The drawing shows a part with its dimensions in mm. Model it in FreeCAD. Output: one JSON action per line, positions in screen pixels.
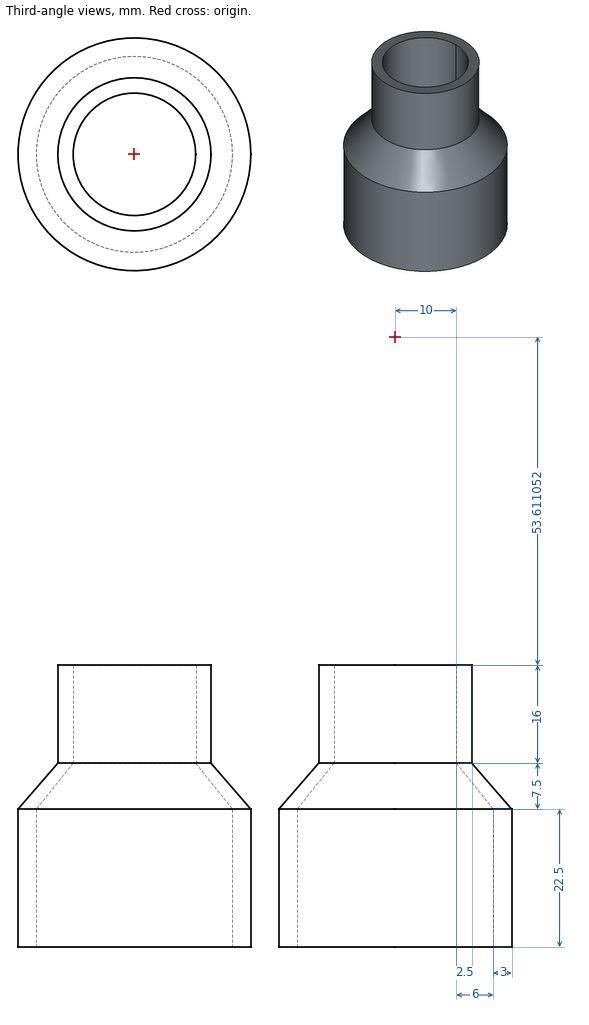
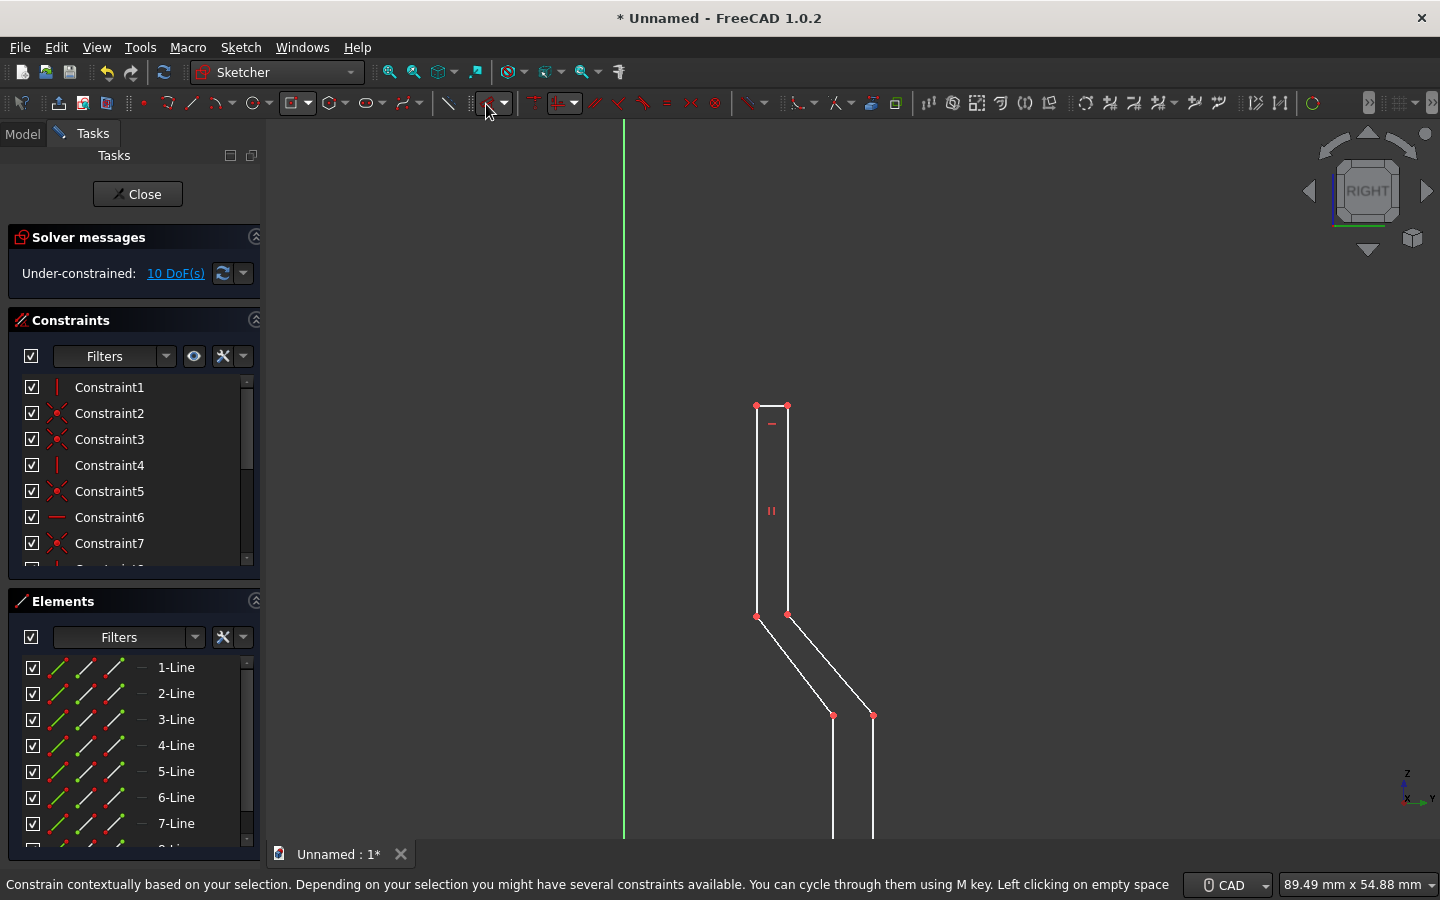
{"action": "scroll", "coordinate": [805, 552], "scroll_direction": "down", "scroll_amount": 5}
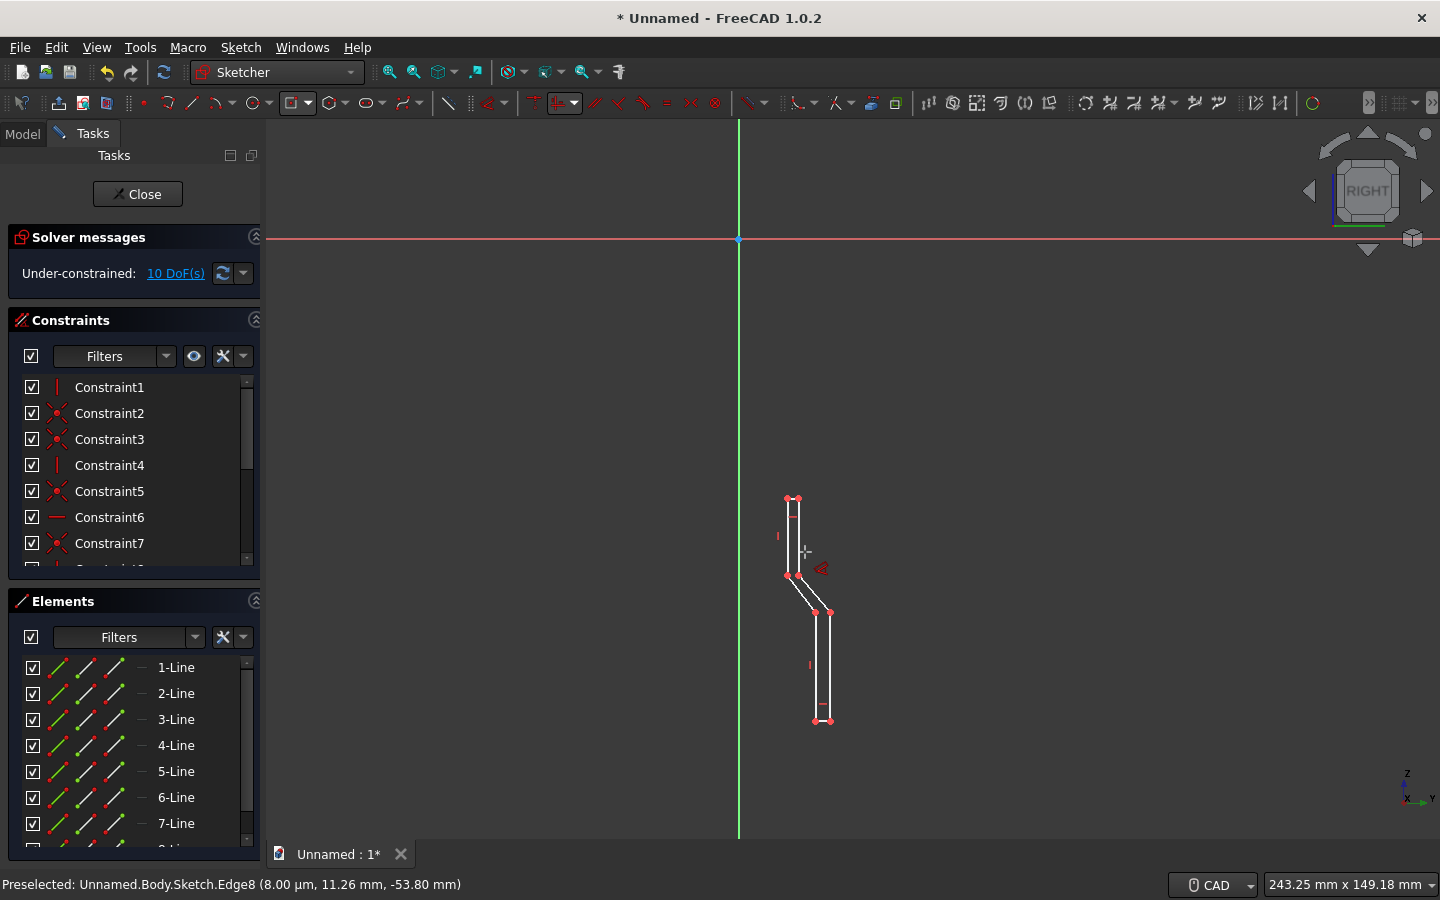
{"action": "scroll", "coordinate": [820, 721], "scroll_direction": "up", "scroll_amount": 6}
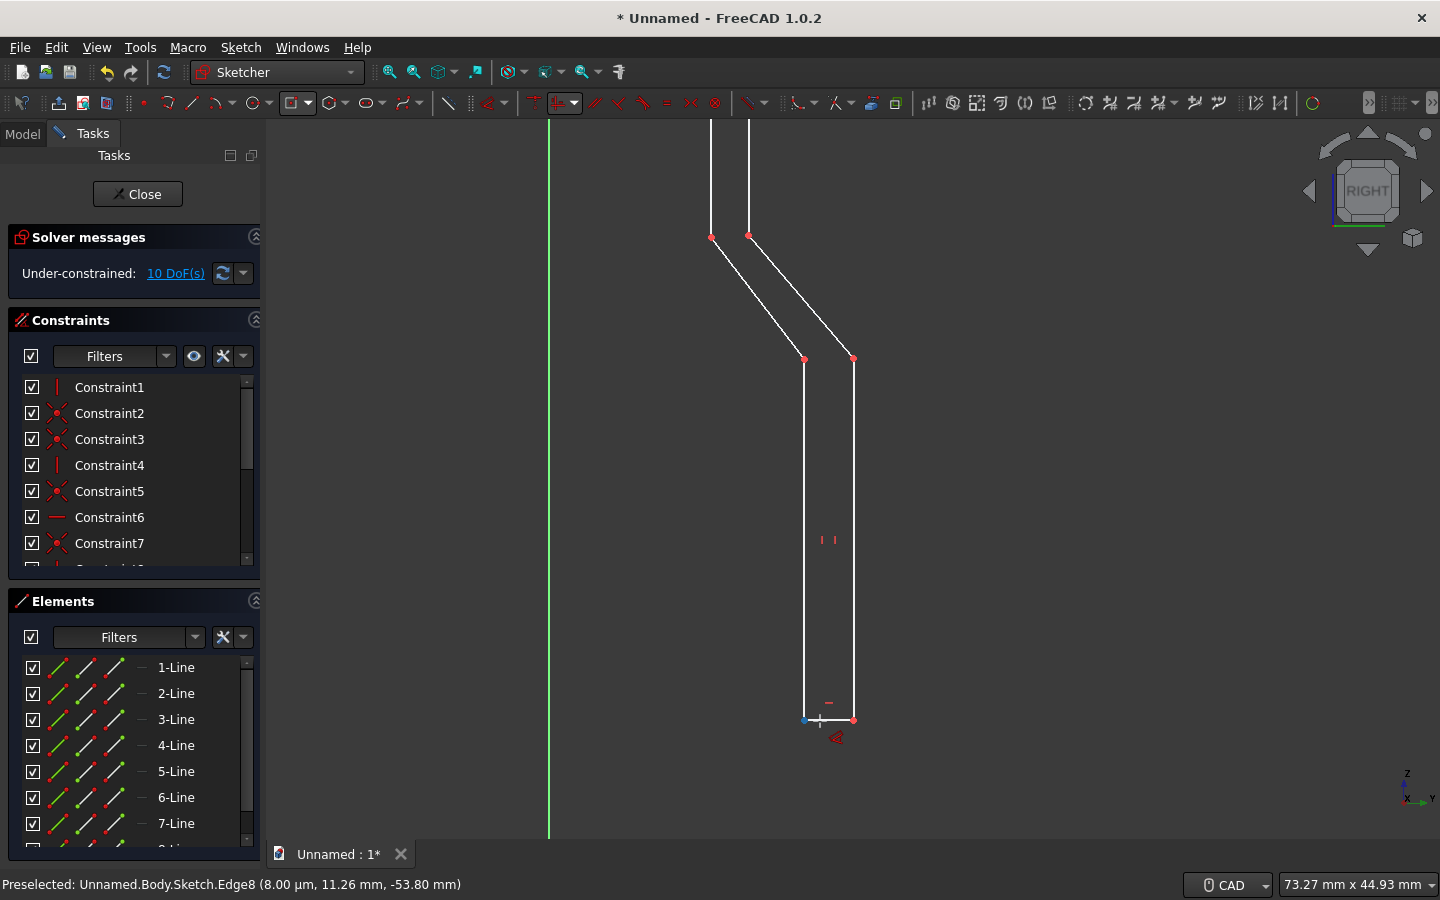
{"action": "left_click", "coordinate": [819, 720]}
{"action": "left_click", "coordinate": [829, 754]}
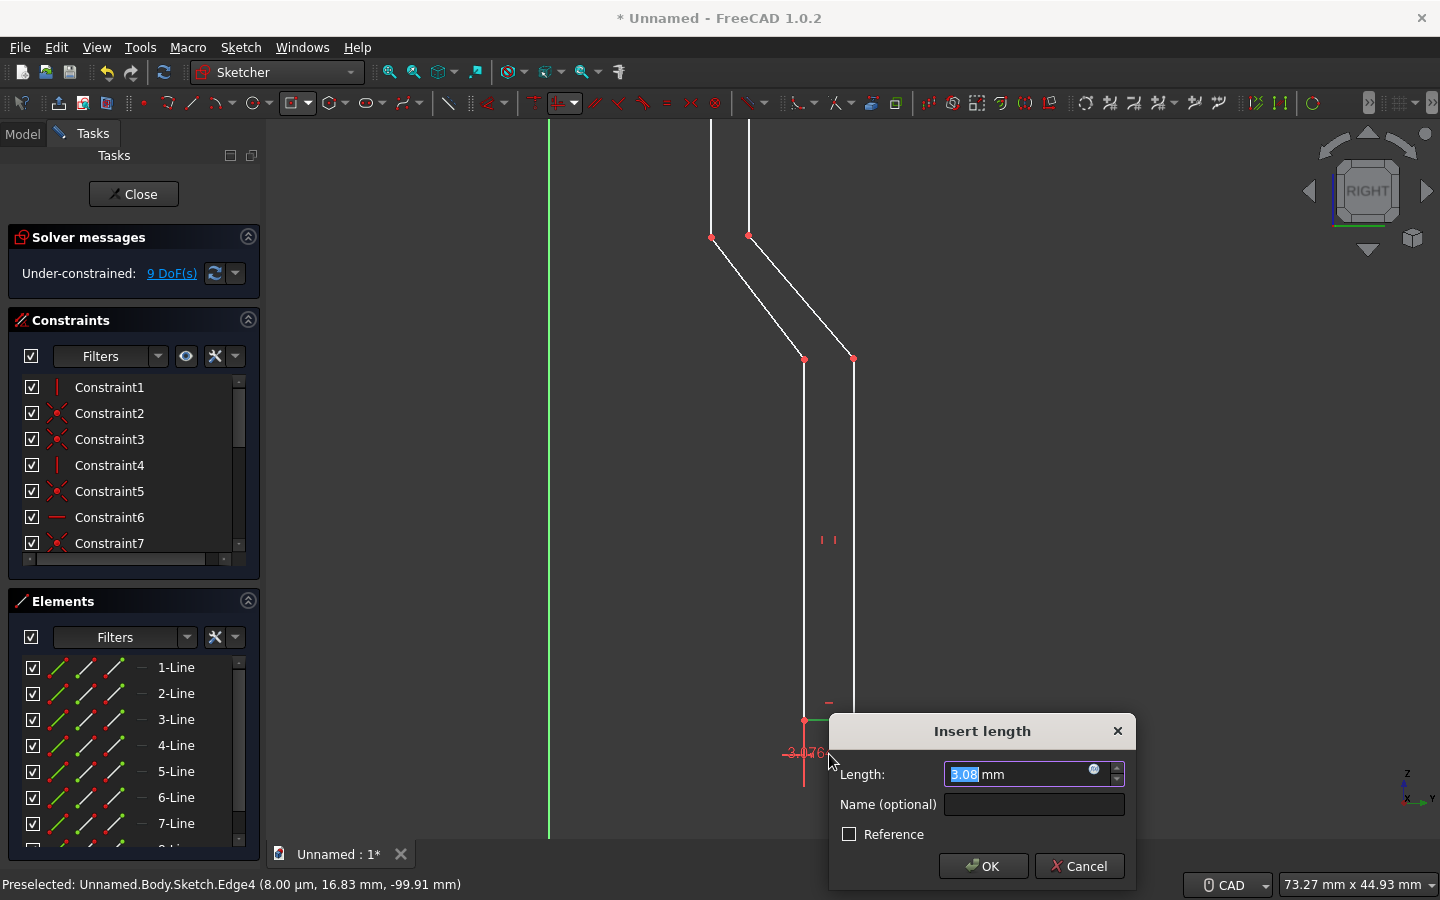
{"action": "type", "text": "3"}
{"action": "key", "text": "Return"}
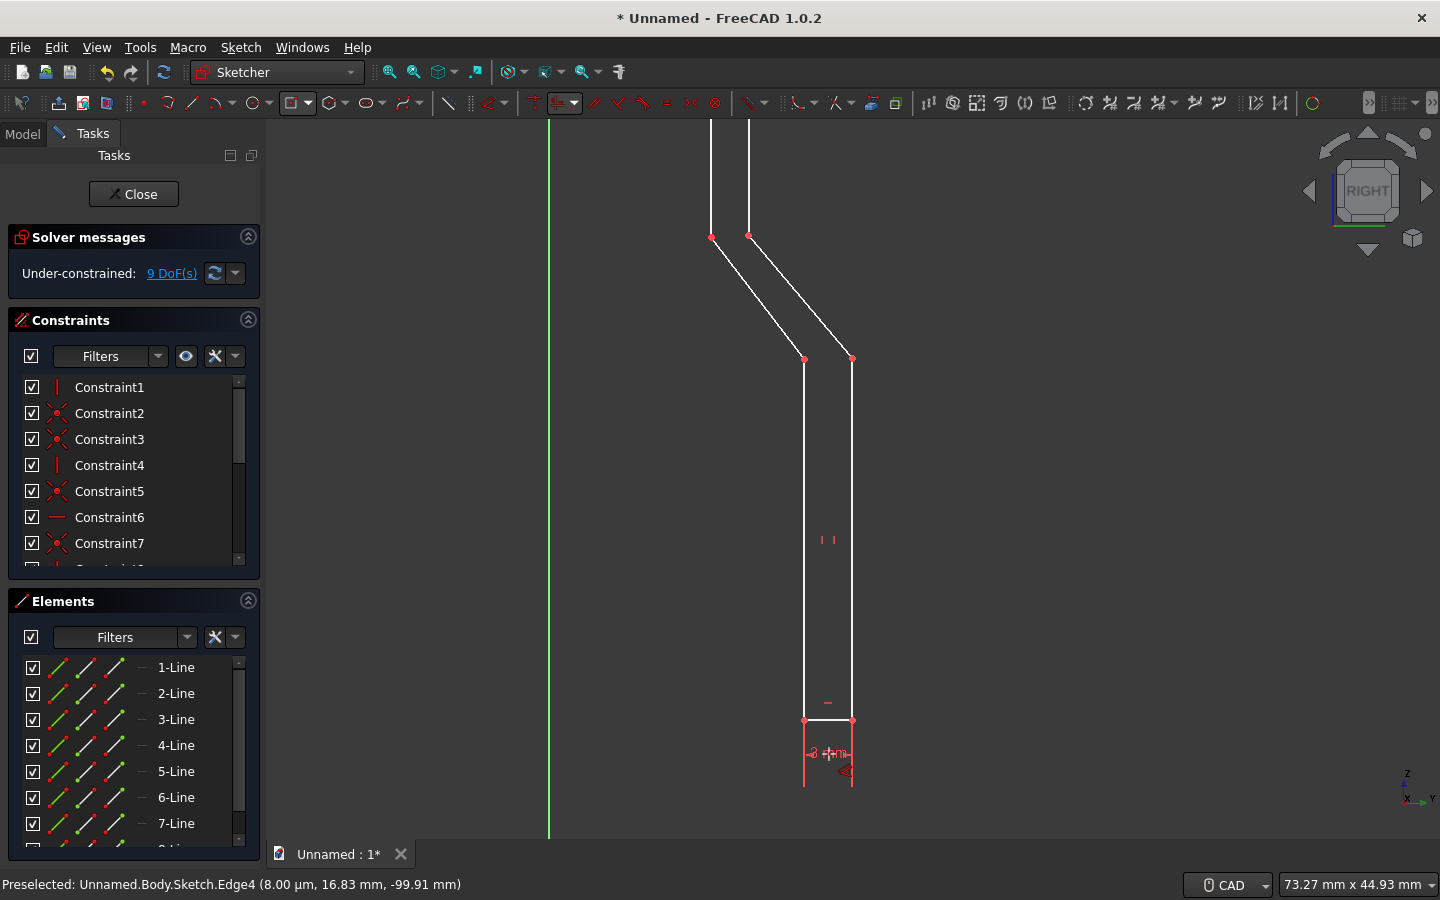
{"action": "left_click", "coordinate": [711, 161]}
{"action": "left_click", "coordinate": [677, 192]}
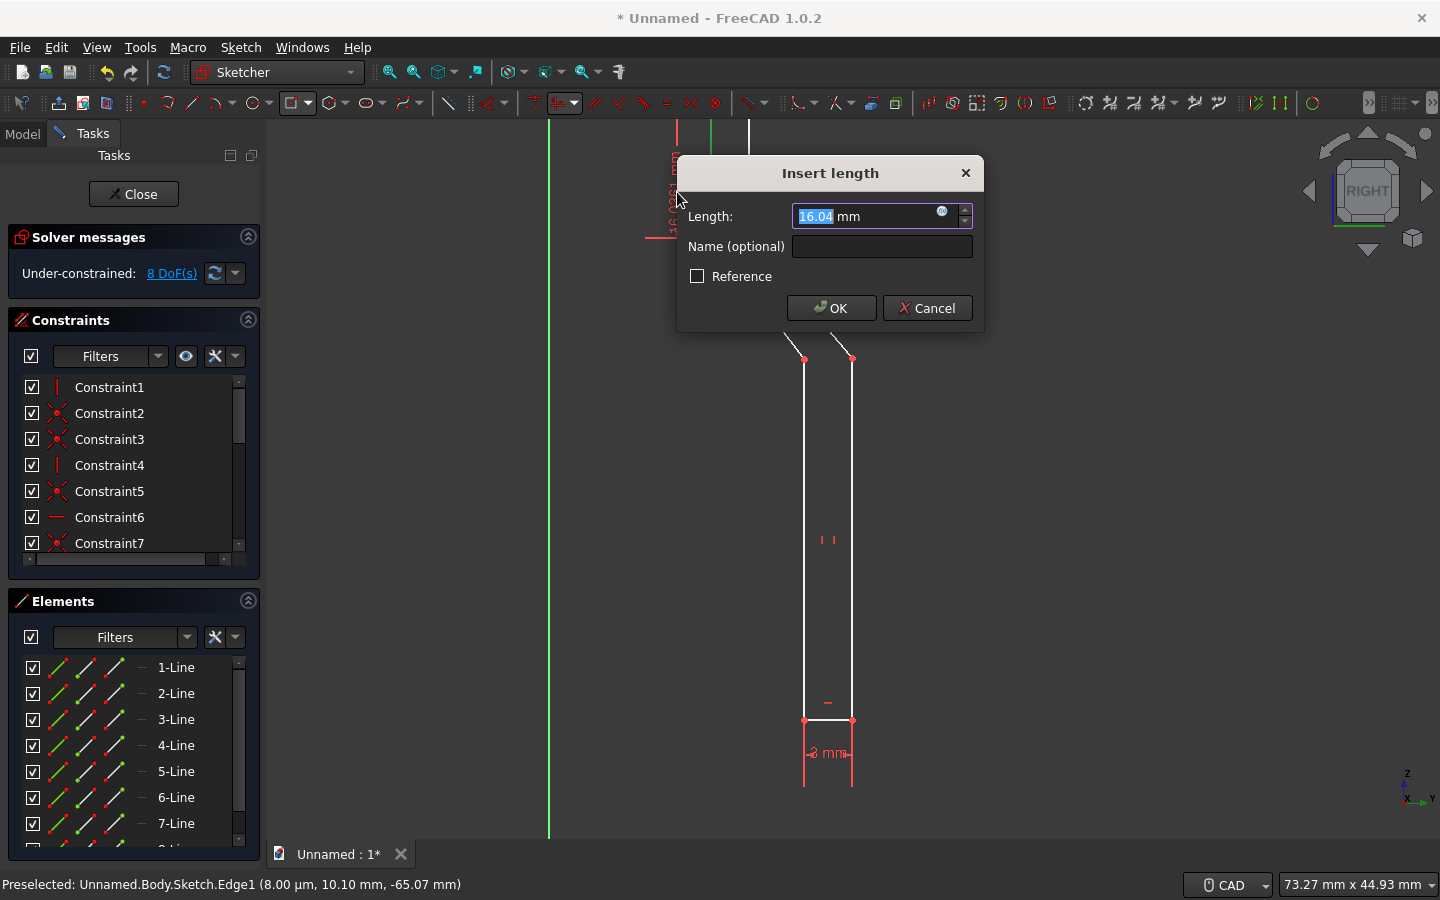
{"action": "type", "text": "16"}
{"action": "key", "text": "Return"}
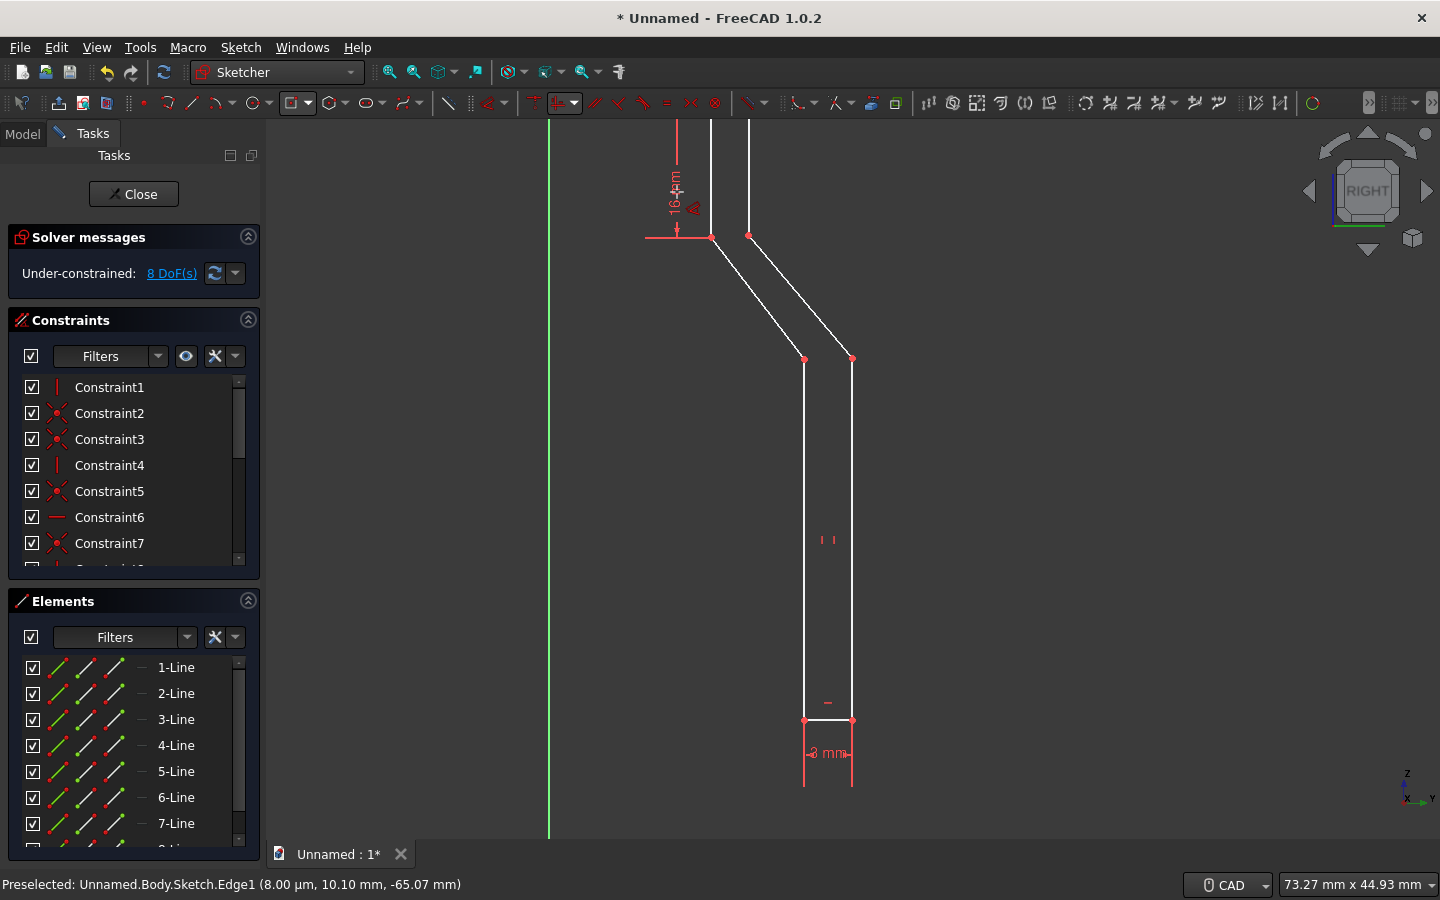
{"action": "left_click", "coordinate": [749, 159]}
{"action": "left_click", "coordinate": [783, 191]}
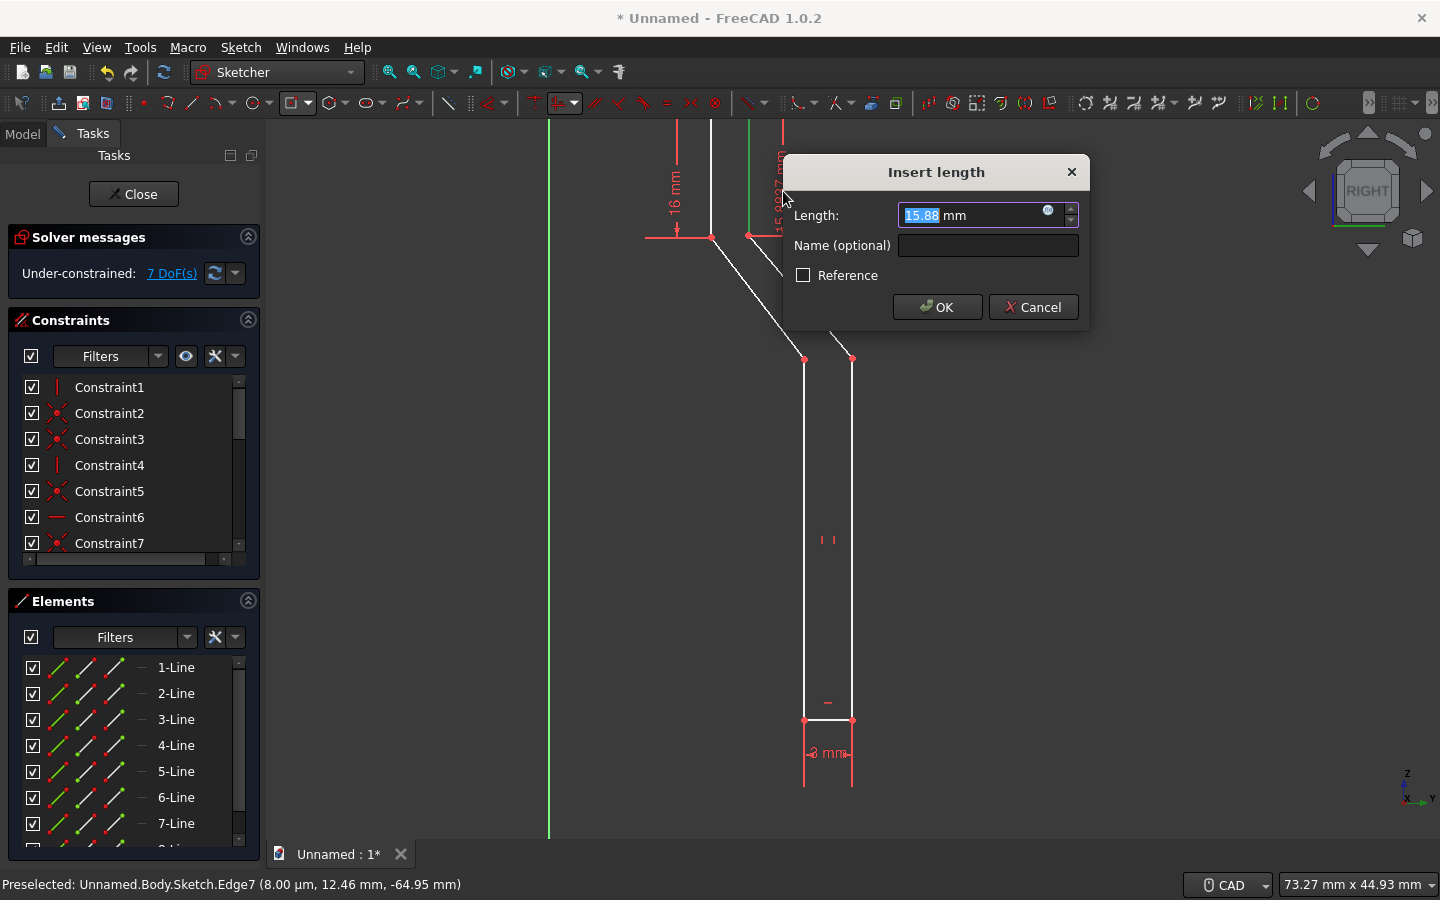
{"action": "type", "text": "16"}
{"action": "key", "text": "Return"}